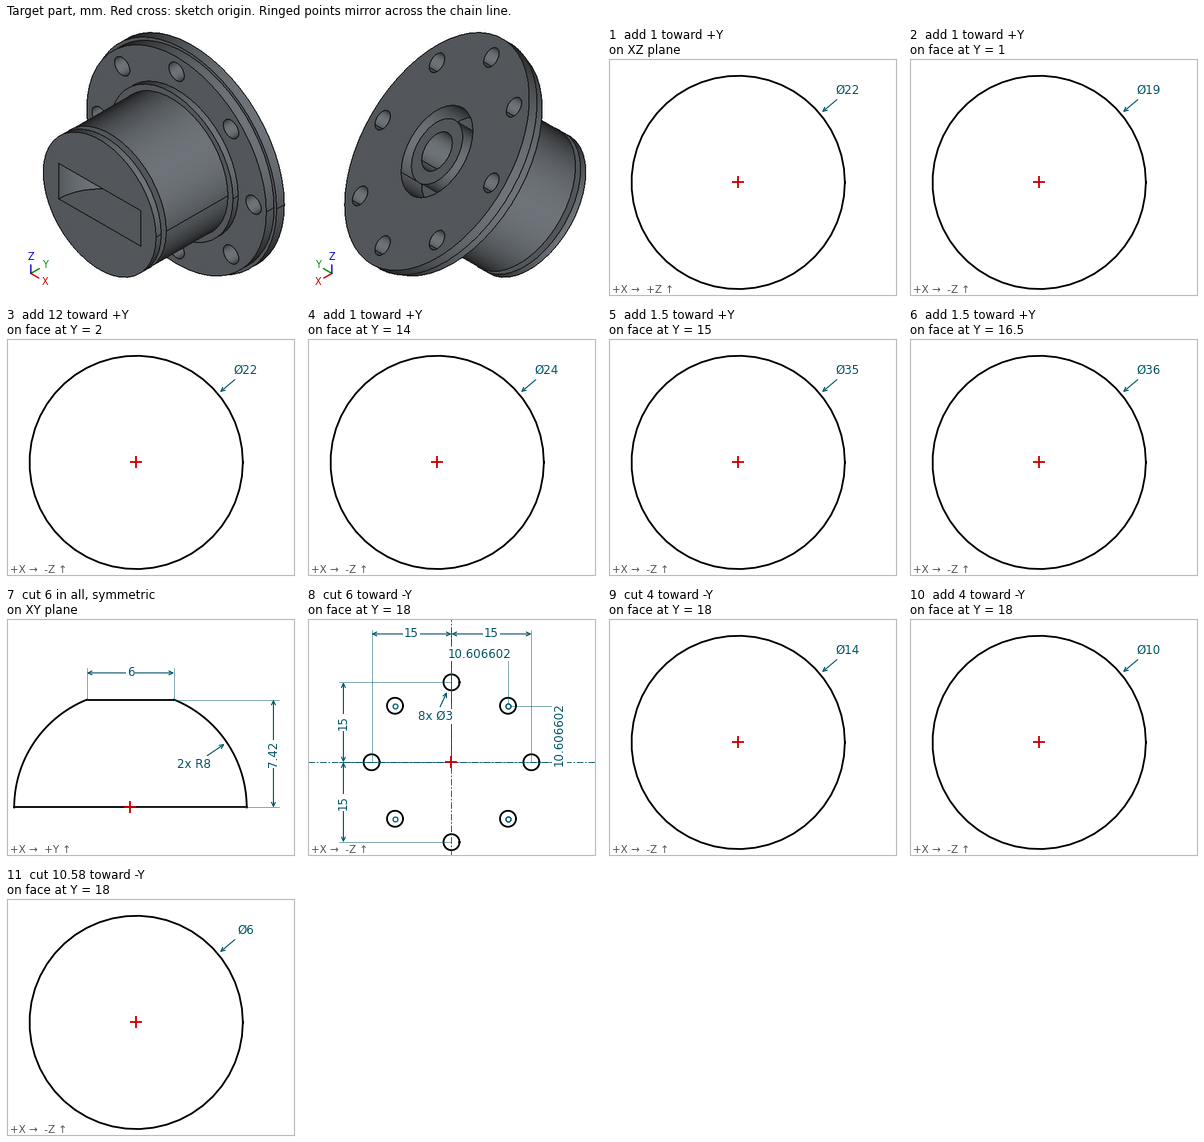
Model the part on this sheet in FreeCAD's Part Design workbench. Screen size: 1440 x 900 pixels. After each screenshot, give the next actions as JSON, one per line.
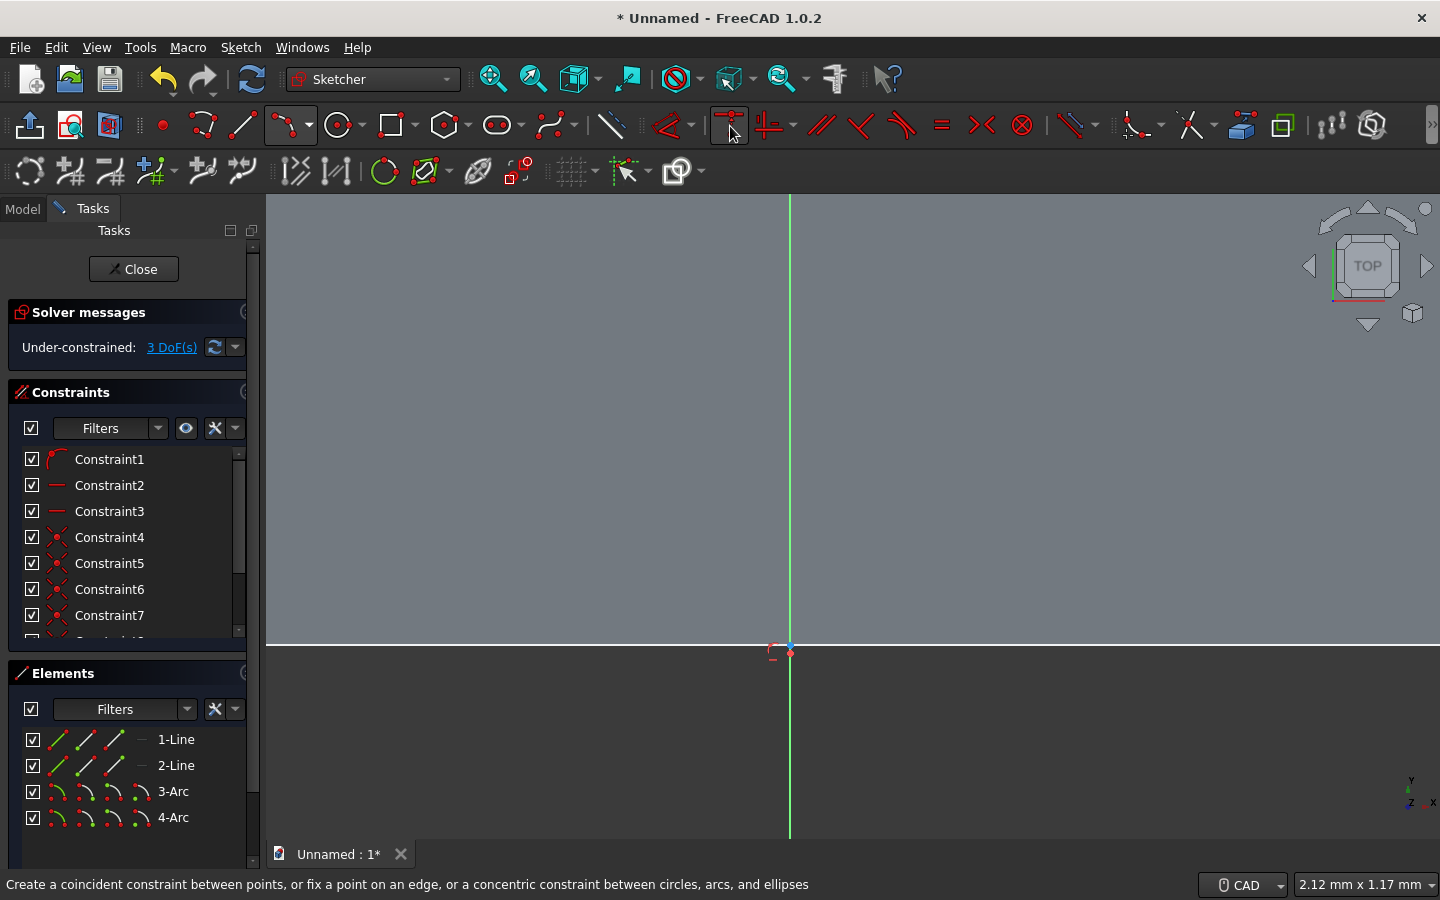
{"action": "left_click", "coordinate": [666, 126]}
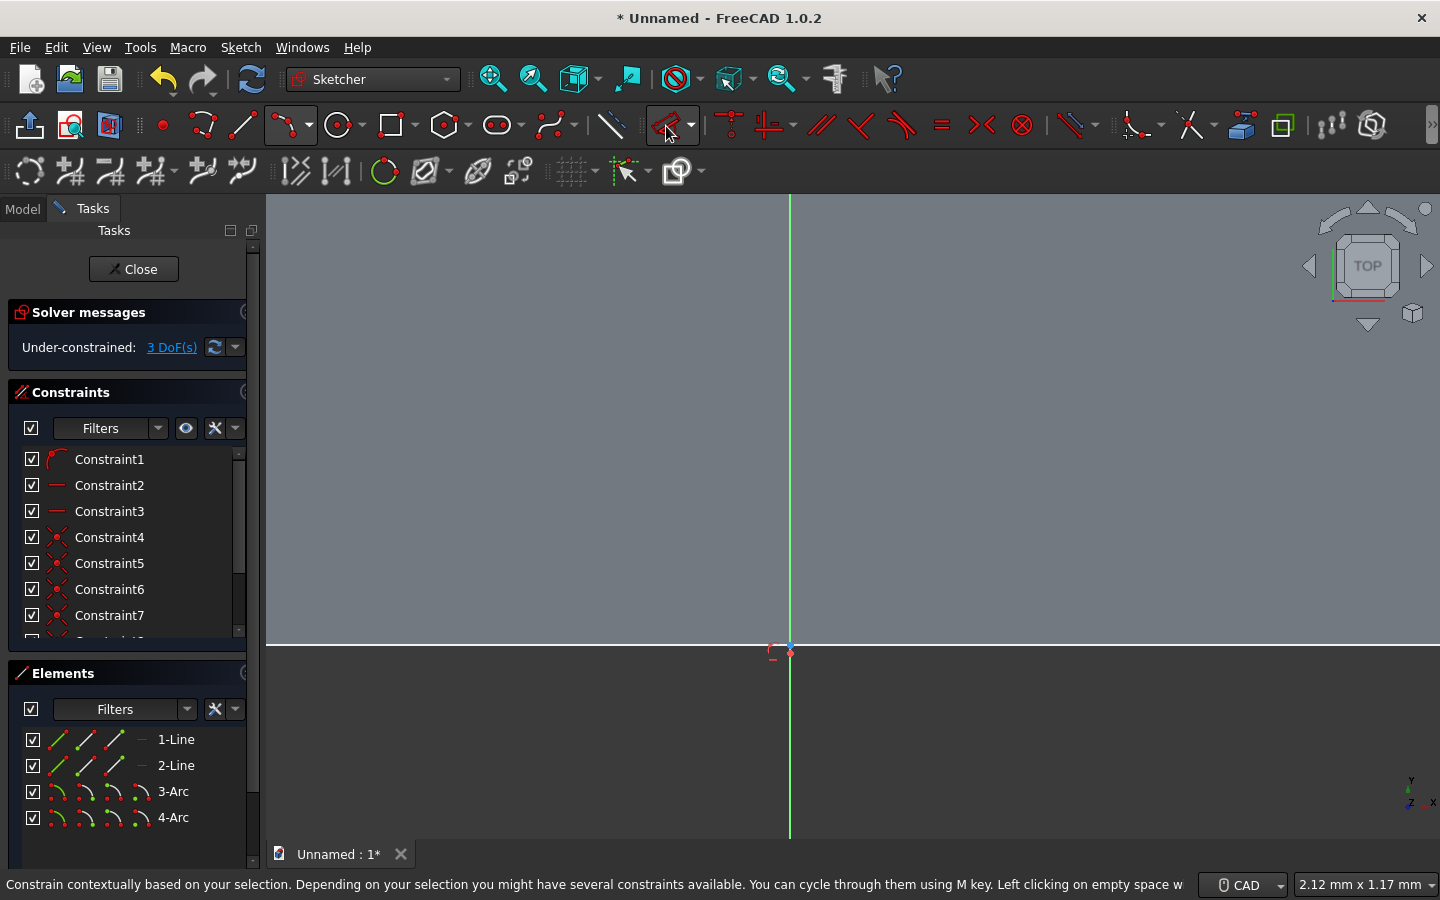
{"action": "scroll", "coordinate": [784, 671], "scroll_direction": "down", "scroll_amount": 13}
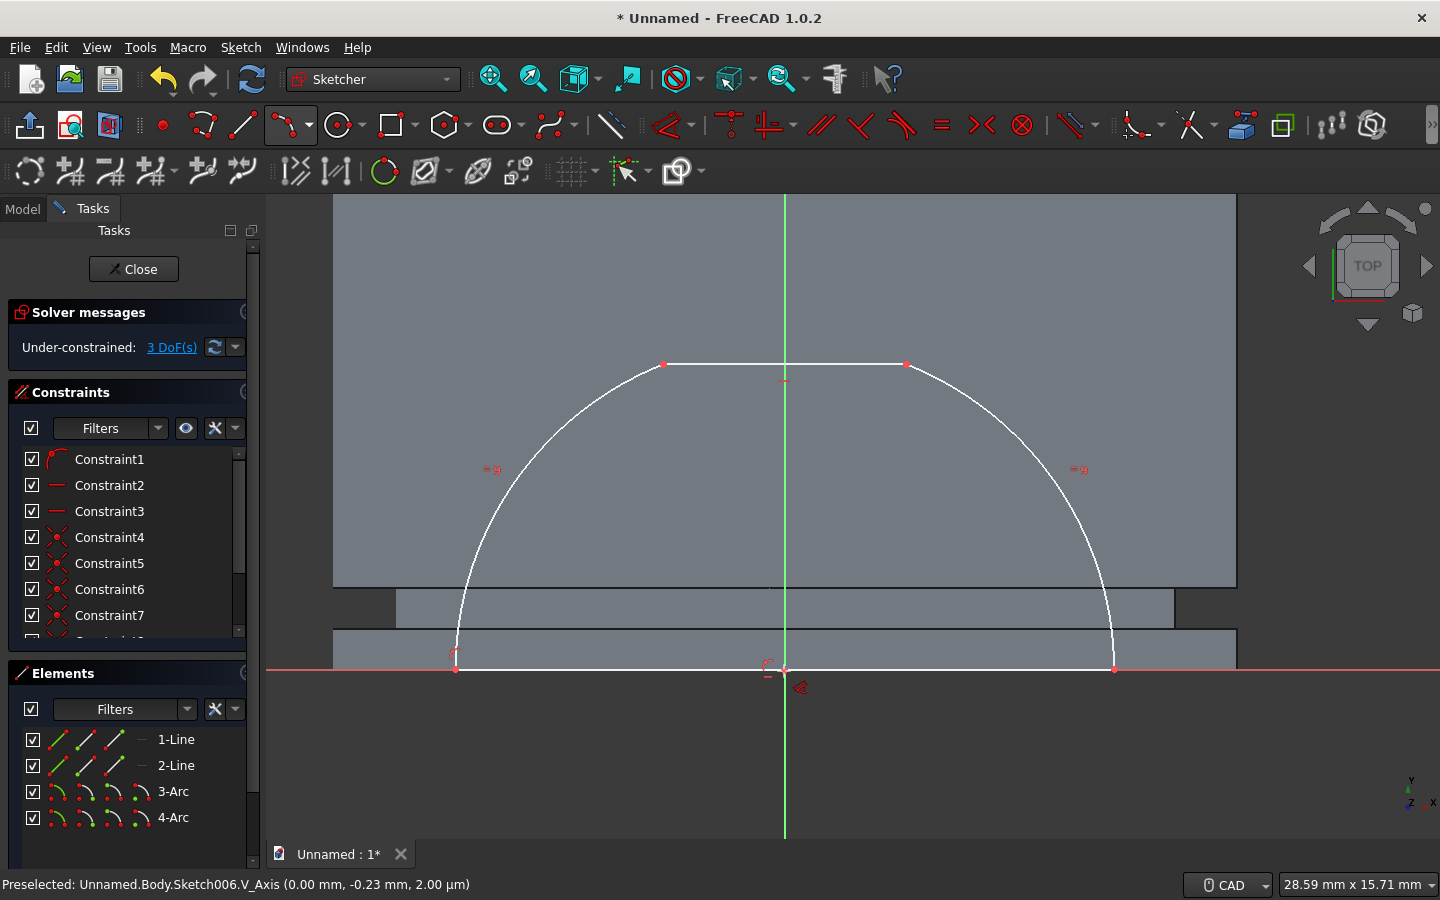
{"action": "left_click", "coordinate": [1093, 555]}
{"action": "left_click", "coordinate": [1123, 544]}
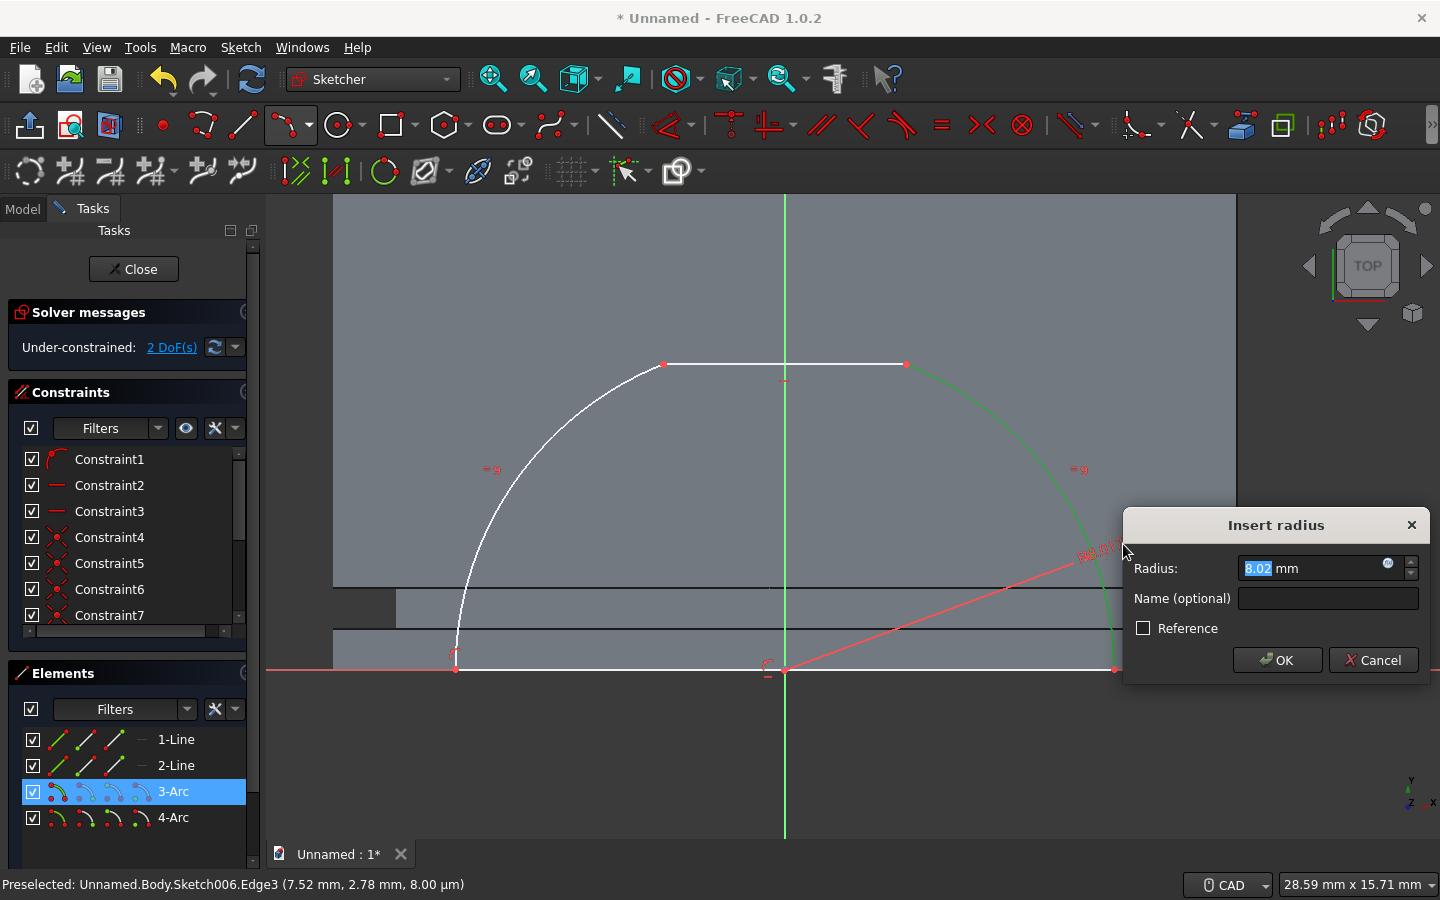
{"action": "type", "text": "8"}
{"action": "key", "text": "Return"}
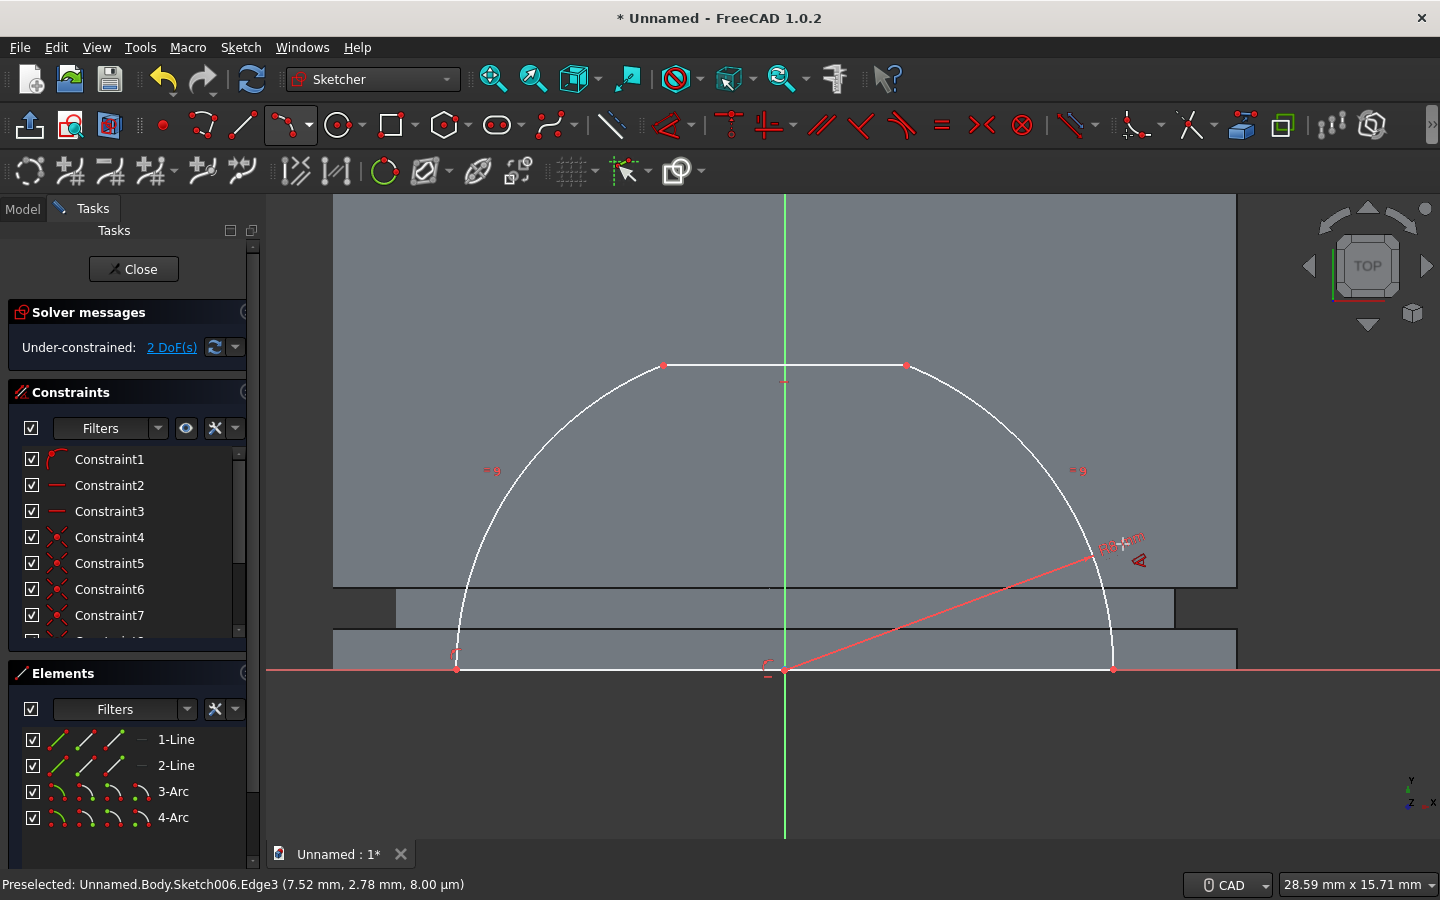
{"action": "left_click", "coordinate": [833, 365]}
{"action": "left_click", "coordinate": [729, 331]}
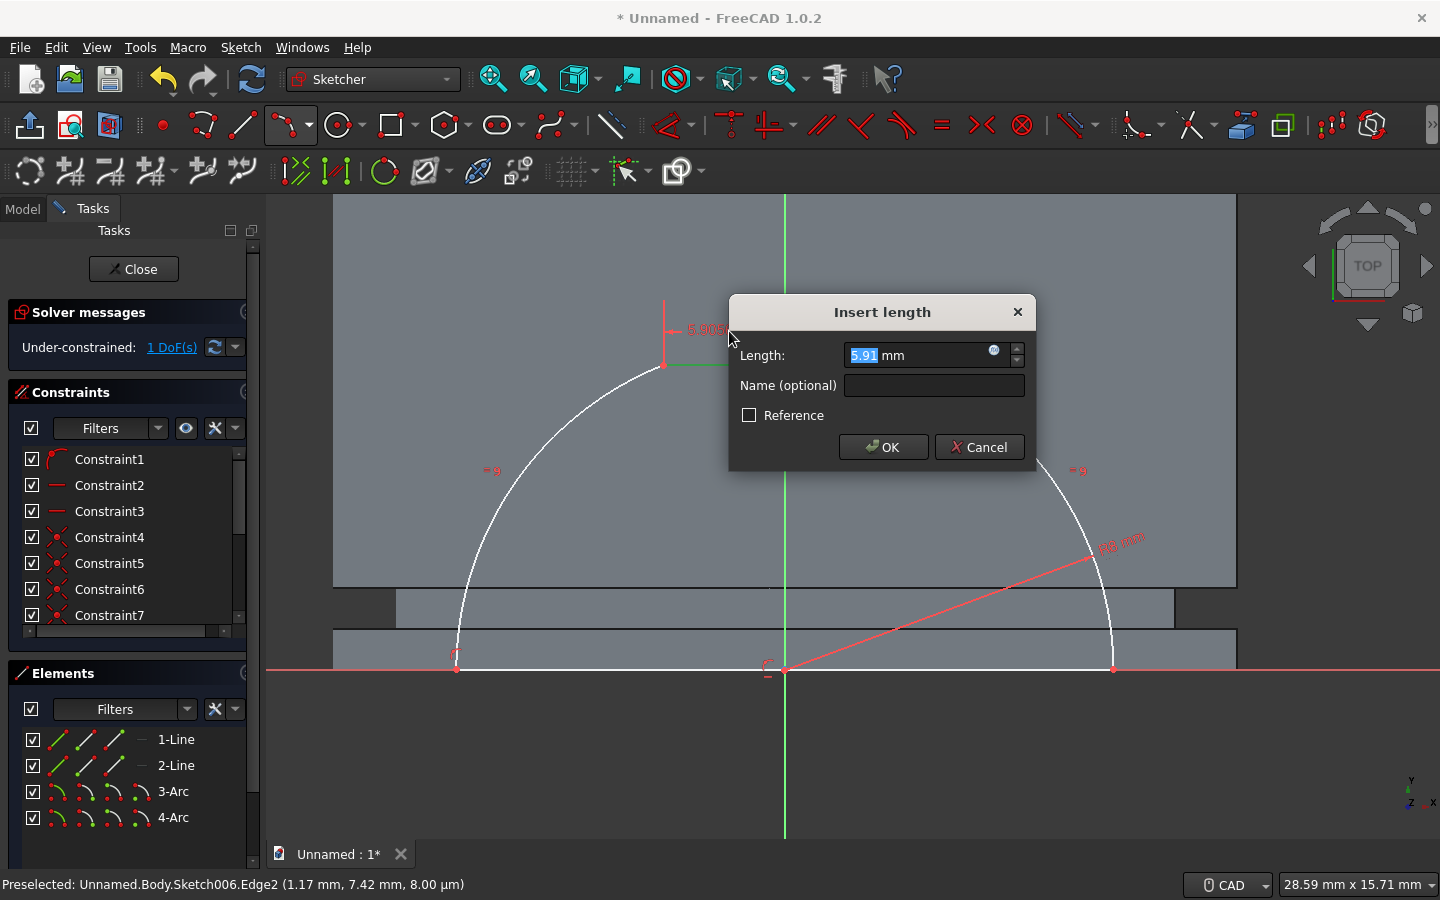
{"action": "type", "text": "6"}
{"action": "key", "text": "Return"}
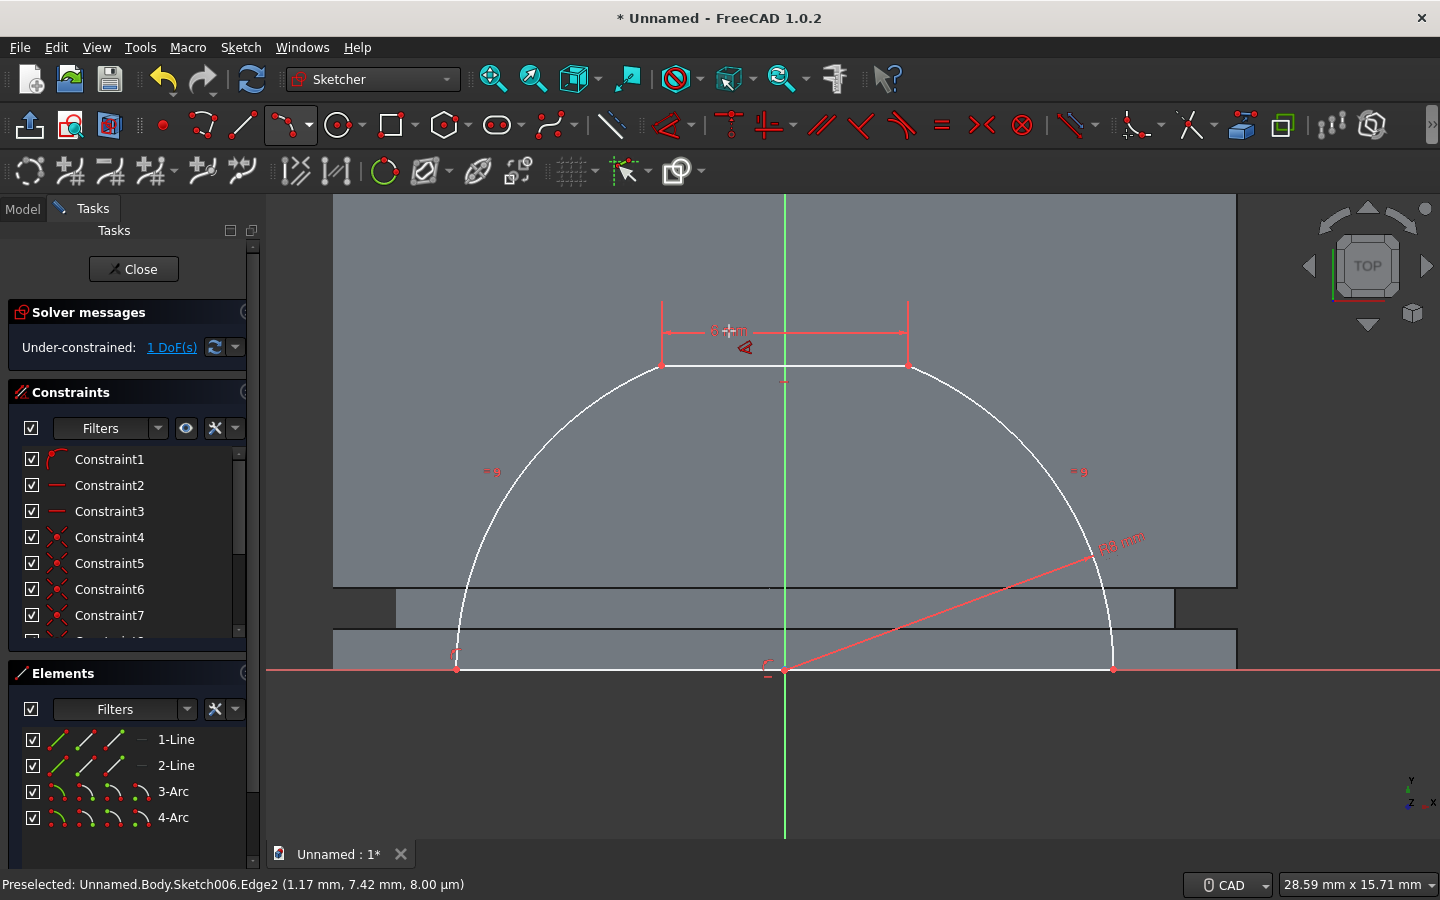
{"action": "left_click", "coordinate": [908, 366]}
{"action": "left_click", "coordinate": [942, 518]}